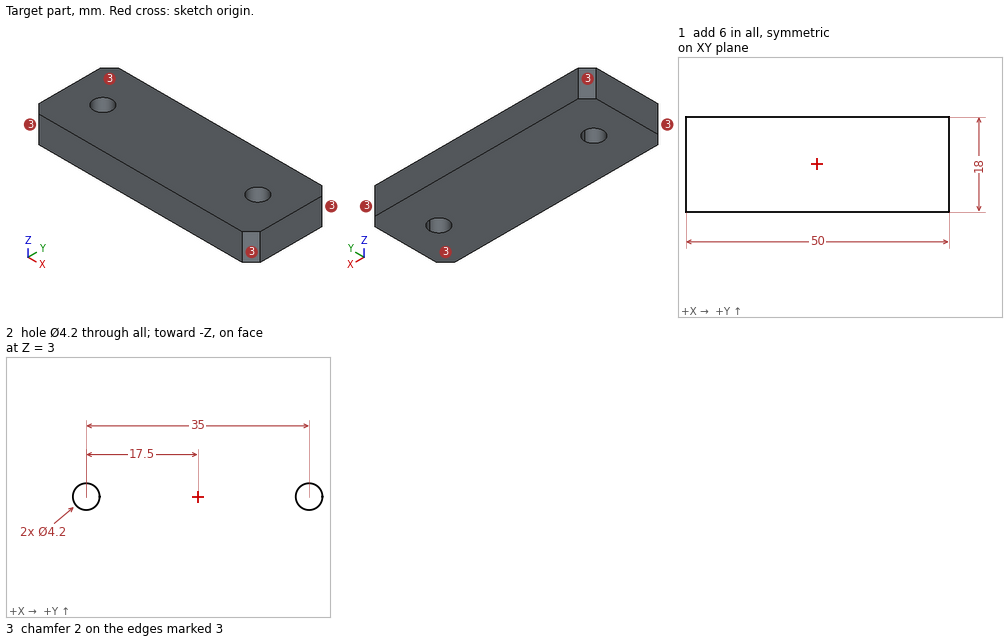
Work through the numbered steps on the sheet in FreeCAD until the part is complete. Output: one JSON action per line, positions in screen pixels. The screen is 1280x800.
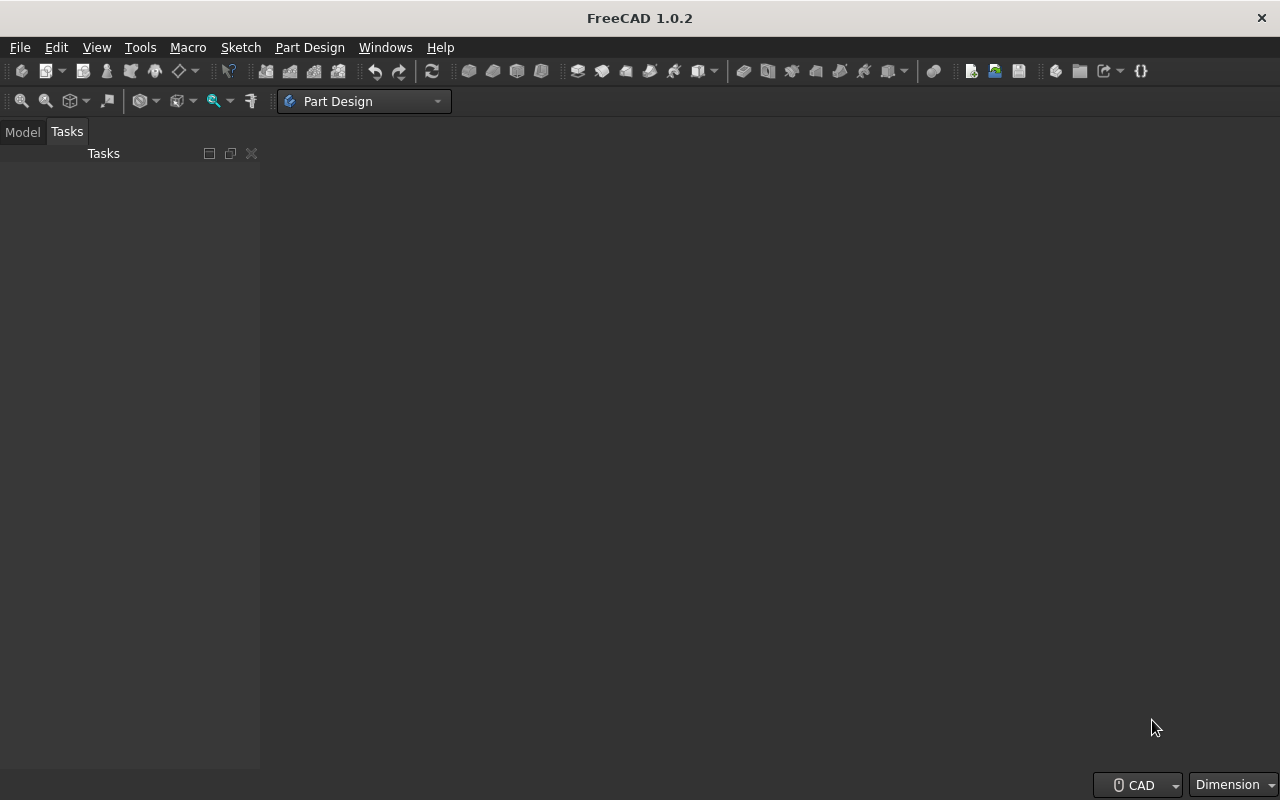
{"action": "key", "text": "ctrl+n"}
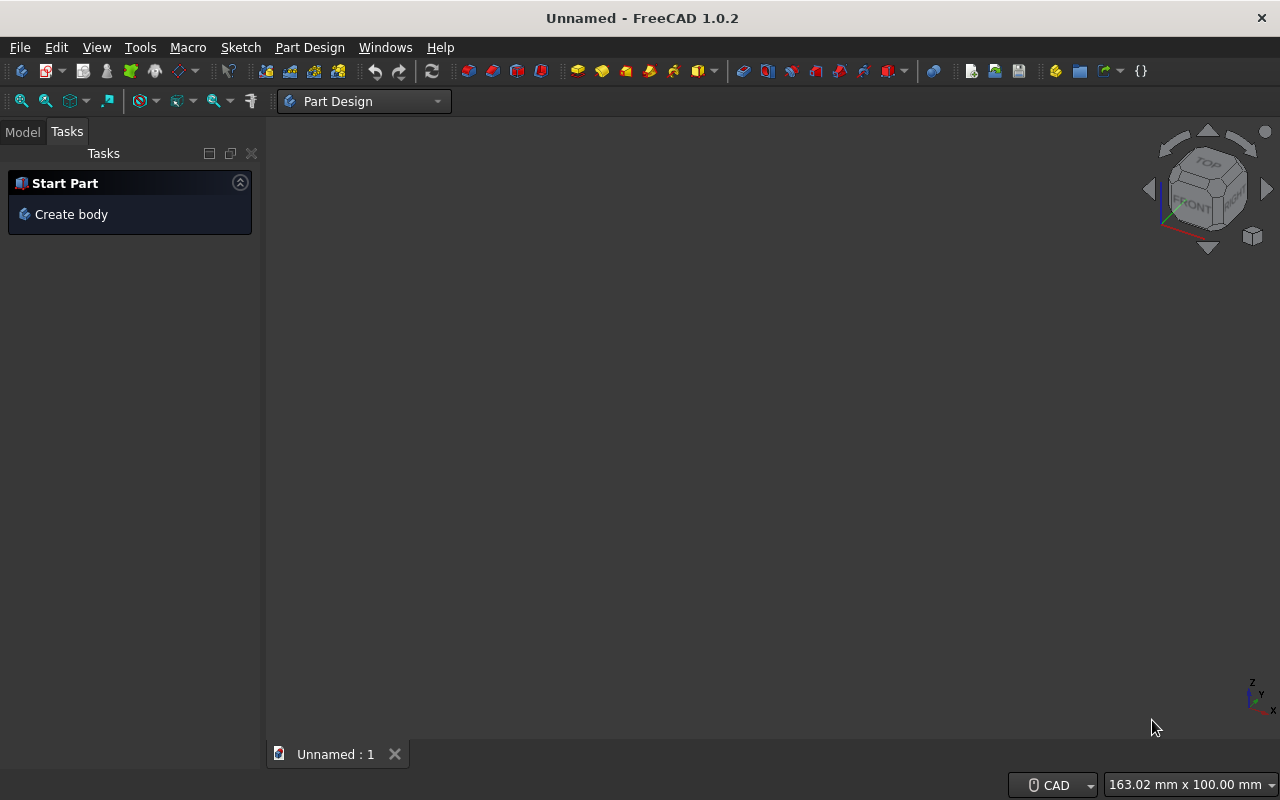
{"action": "left_click", "coordinate": [46, 72]}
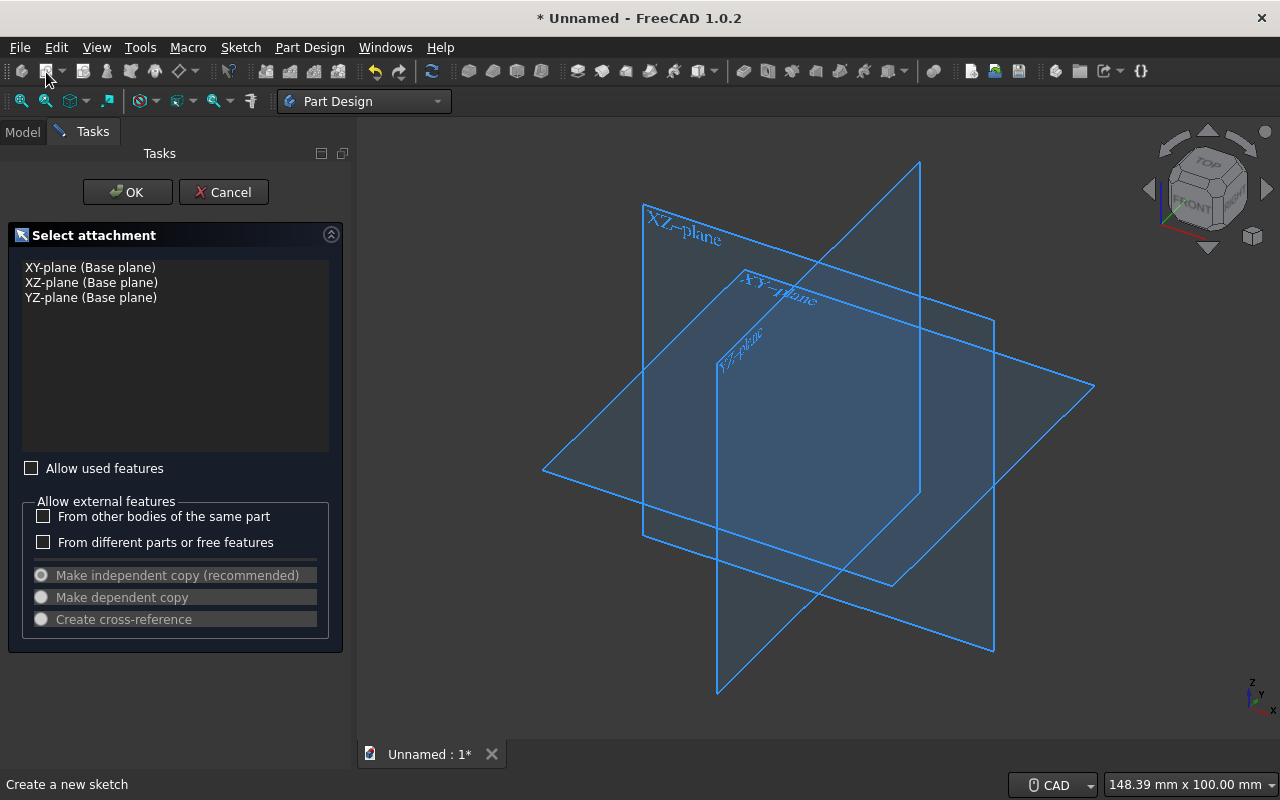
{"action": "left_click", "coordinate": [82, 268]}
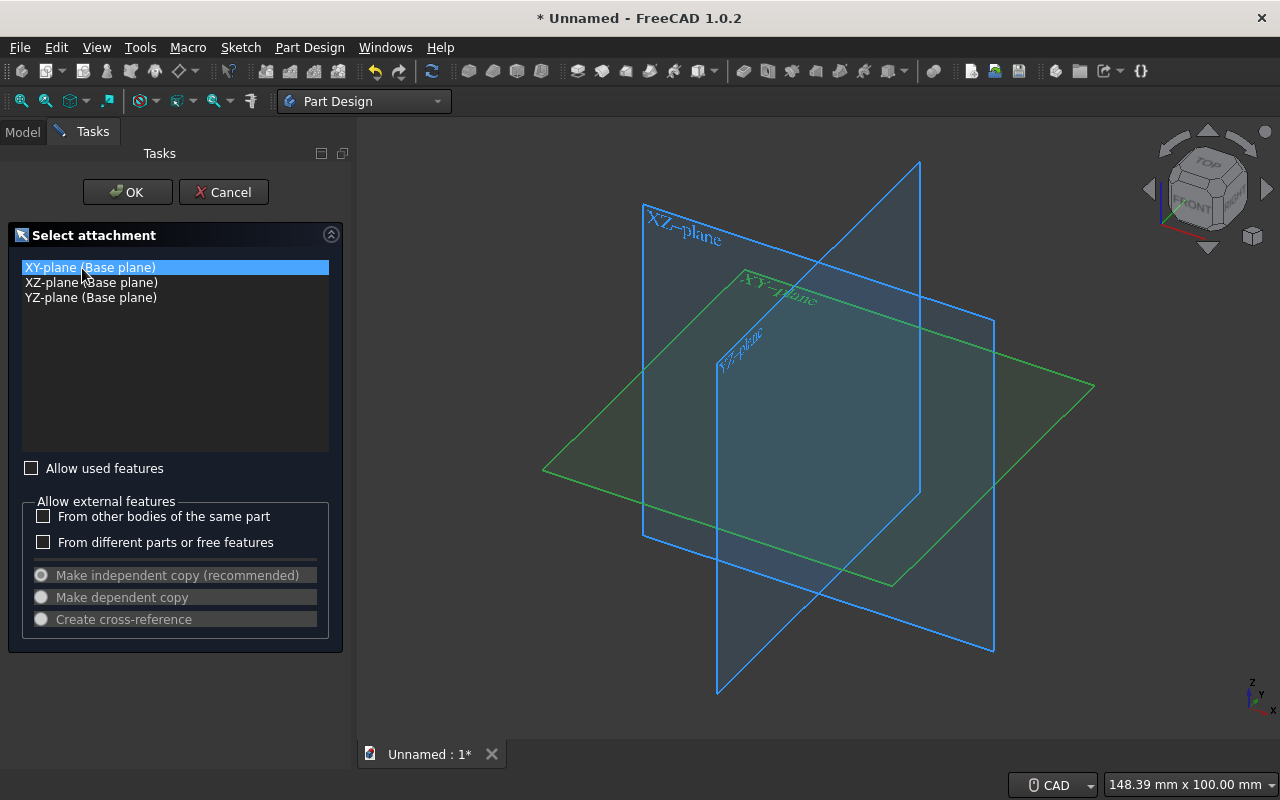
{"action": "left_click", "coordinate": [128, 192]}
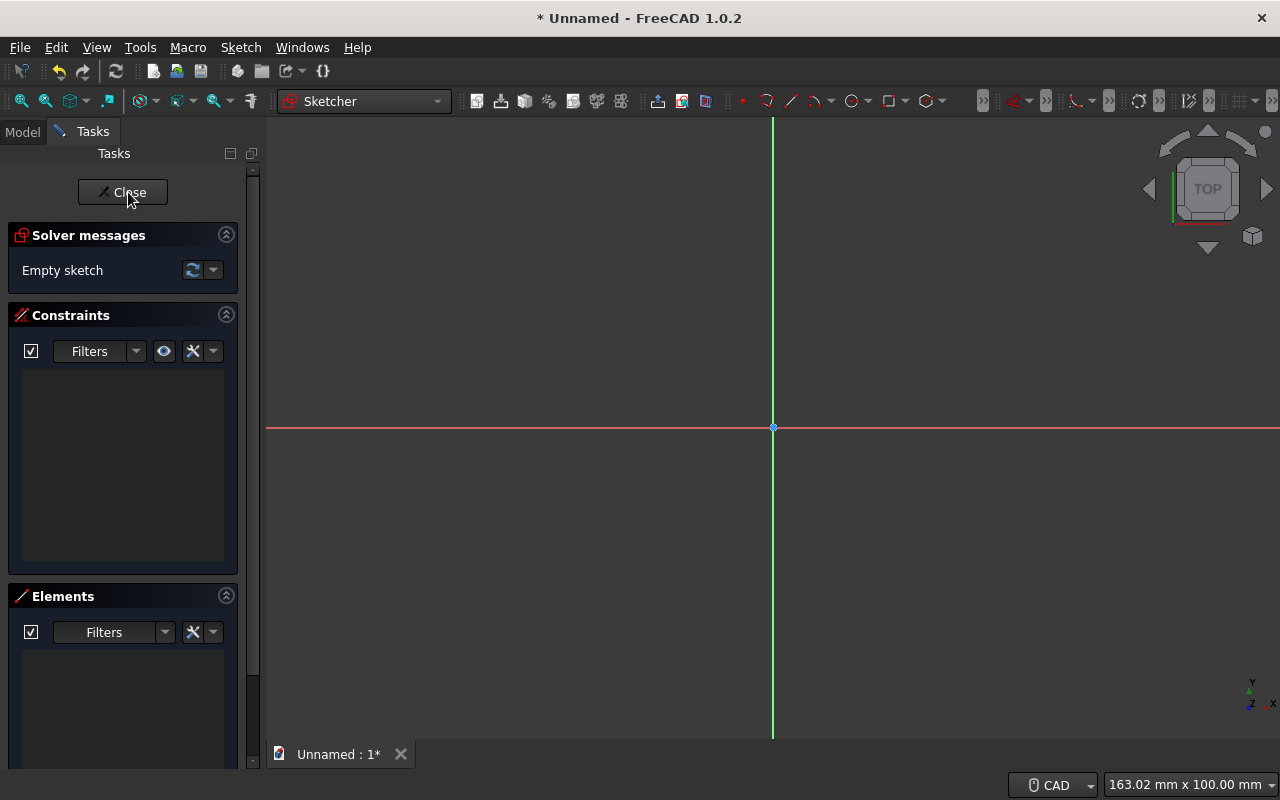
{"action": "scroll", "coordinate": [856, 428], "scroll_direction": "up", "scroll_amount": 3}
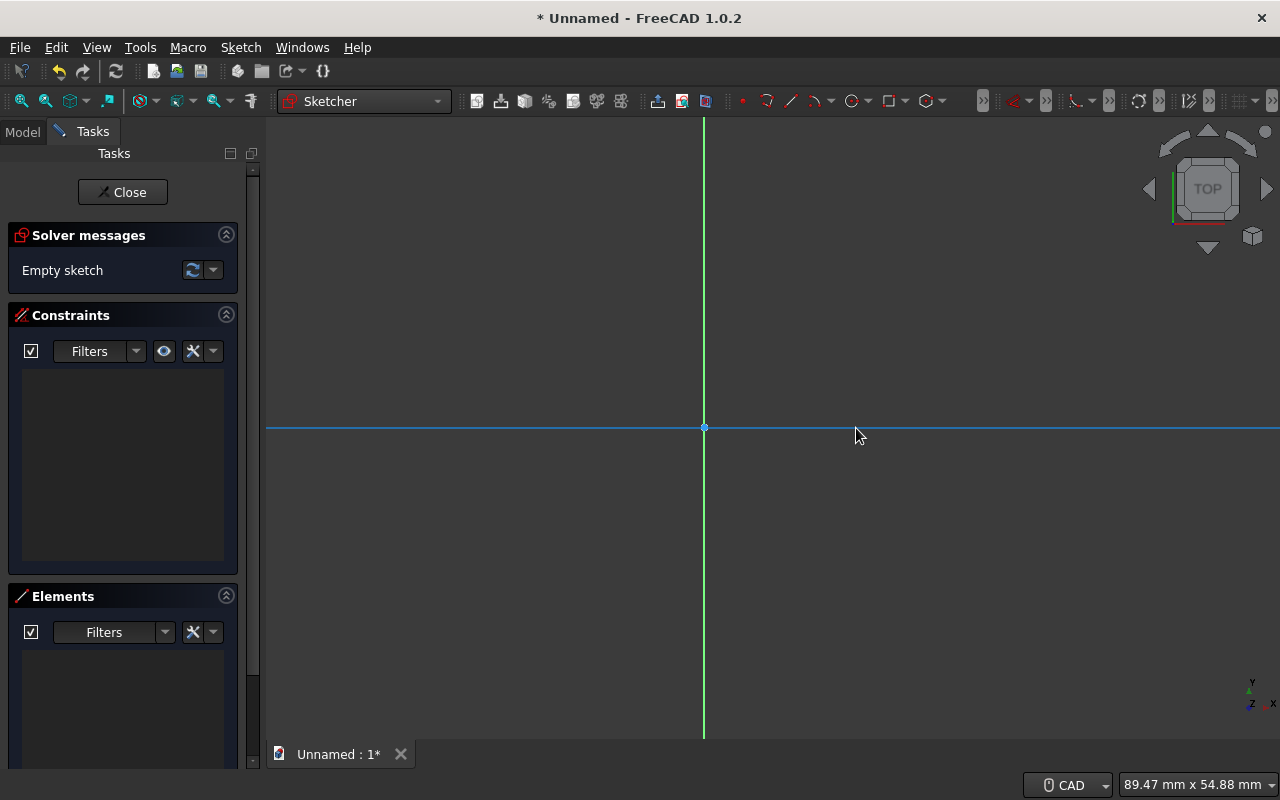
{"action": "key", "text": "g v"}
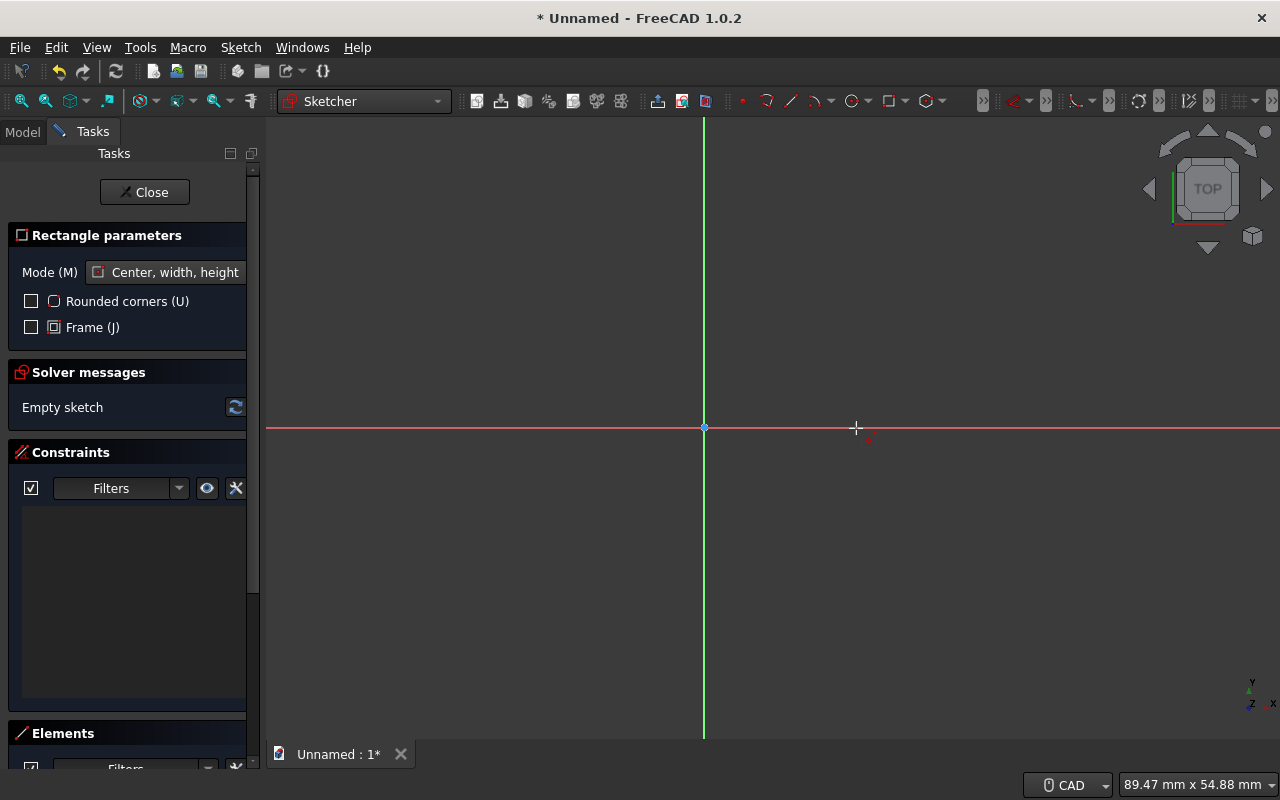
{"action": "left_click", "coordinate": [704, 428]}
{"action": "left_click", "coordinate": [988, 326]}
{"action": "key", "text": "Escape"}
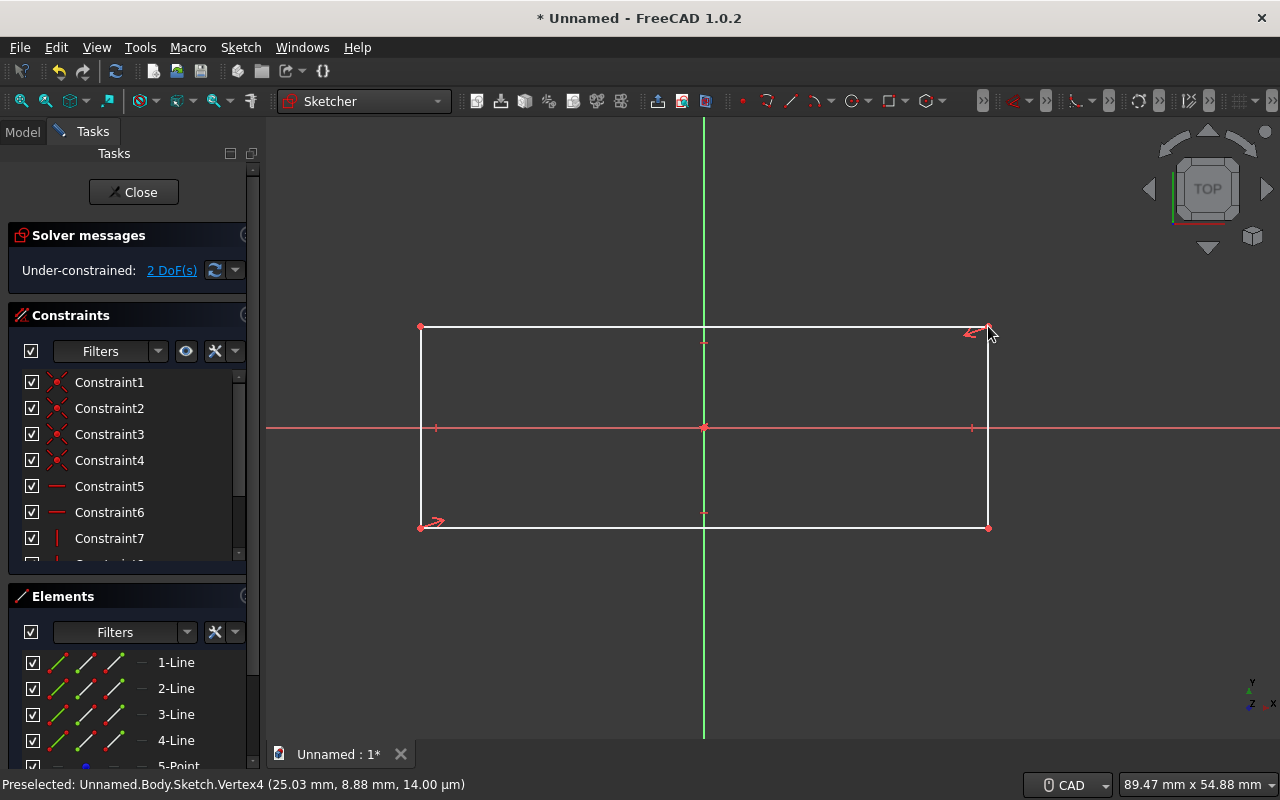
{"action": "left_click", "coordinate": [1014, 102]}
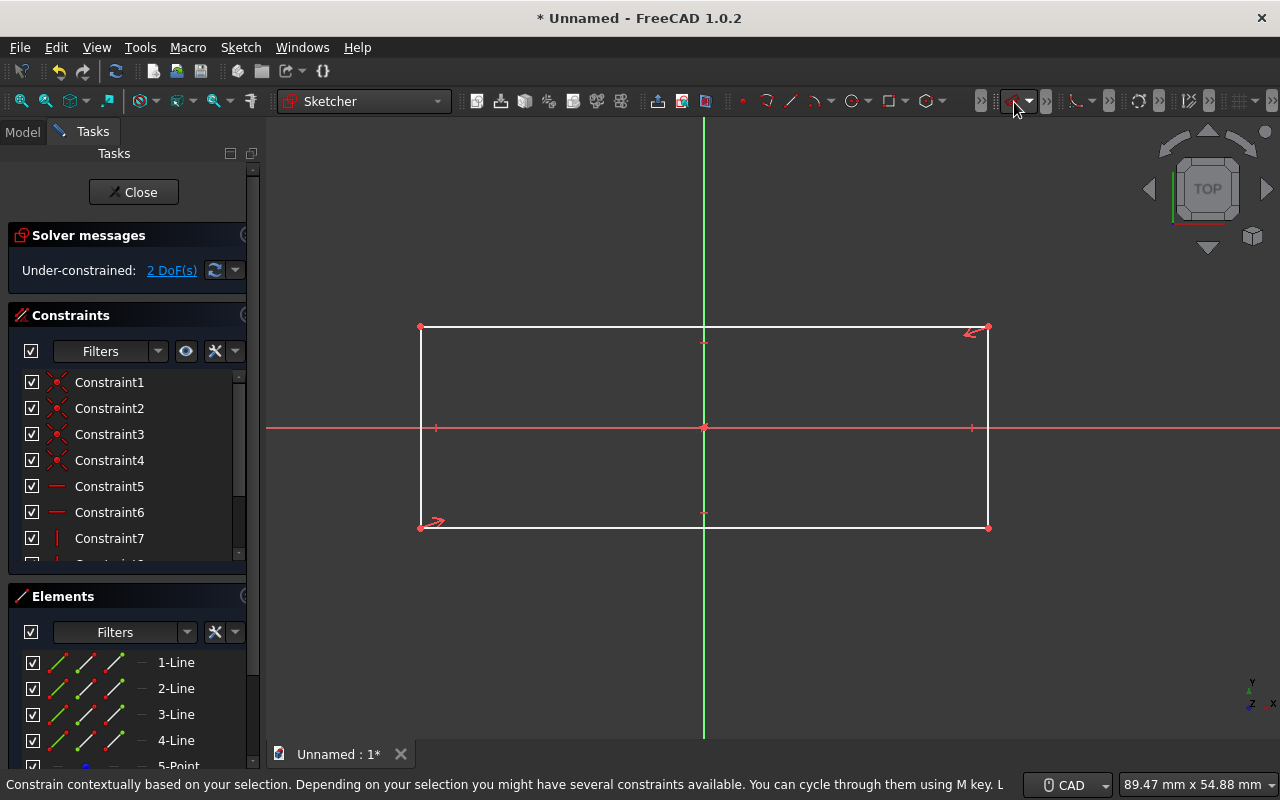
{"action": "left_click", "coordinate": [591, 528]}
{"action": "left_click", "coordinate": [574, 562]}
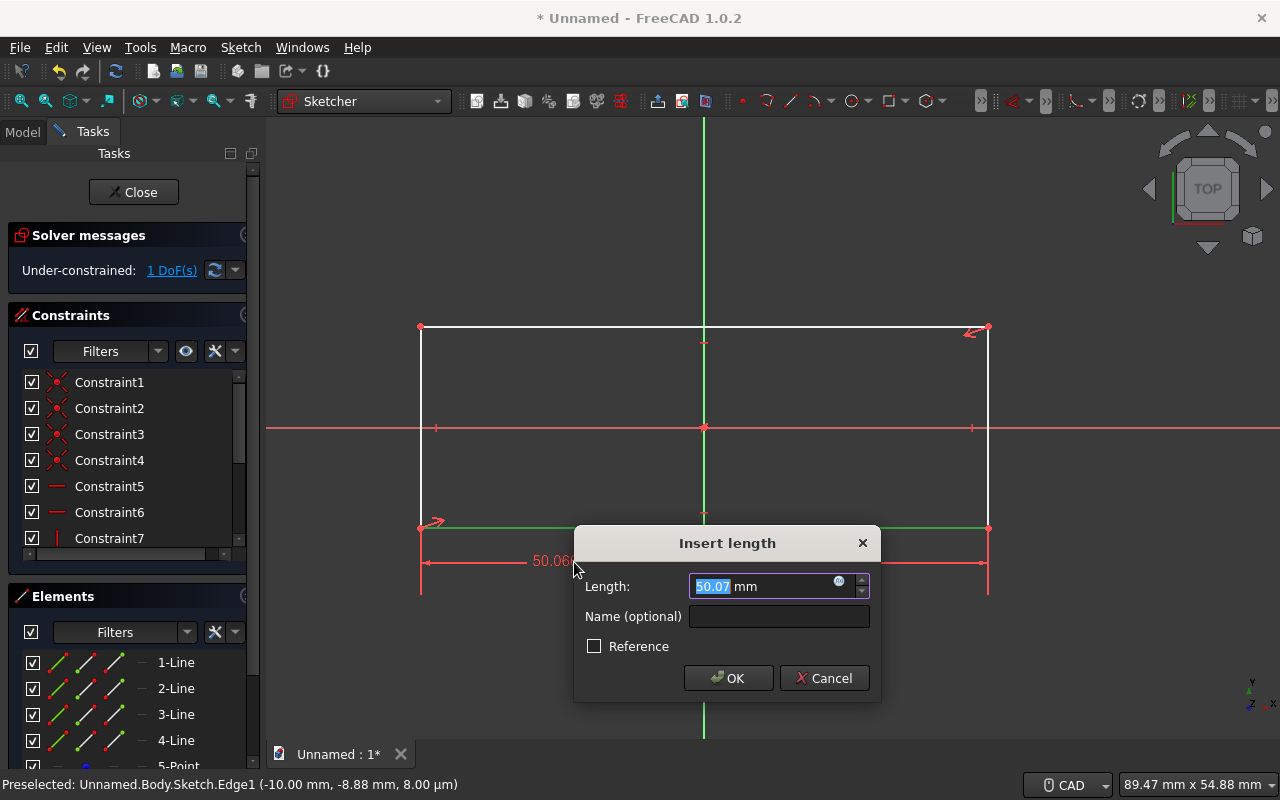
{"action": "type", "text": "50"}
{"action": "key", "text": "Return"}